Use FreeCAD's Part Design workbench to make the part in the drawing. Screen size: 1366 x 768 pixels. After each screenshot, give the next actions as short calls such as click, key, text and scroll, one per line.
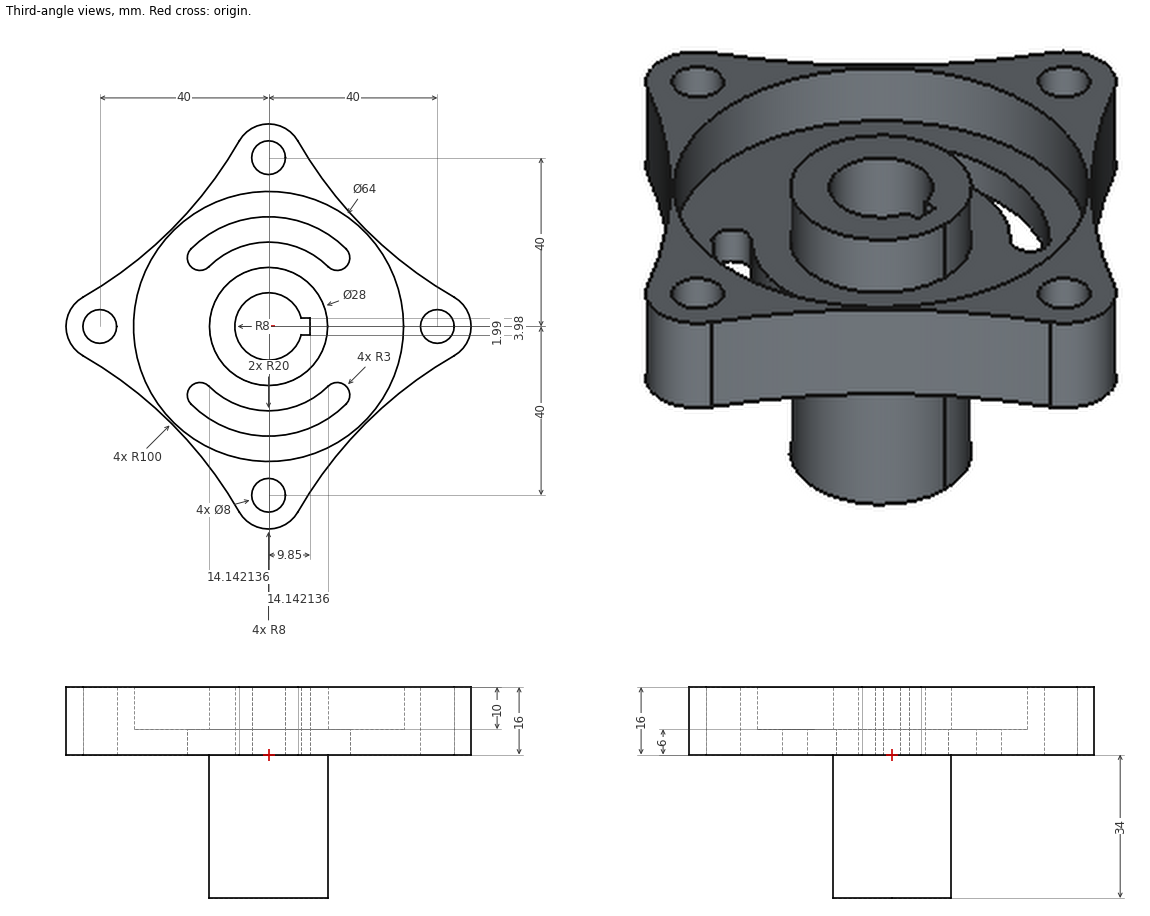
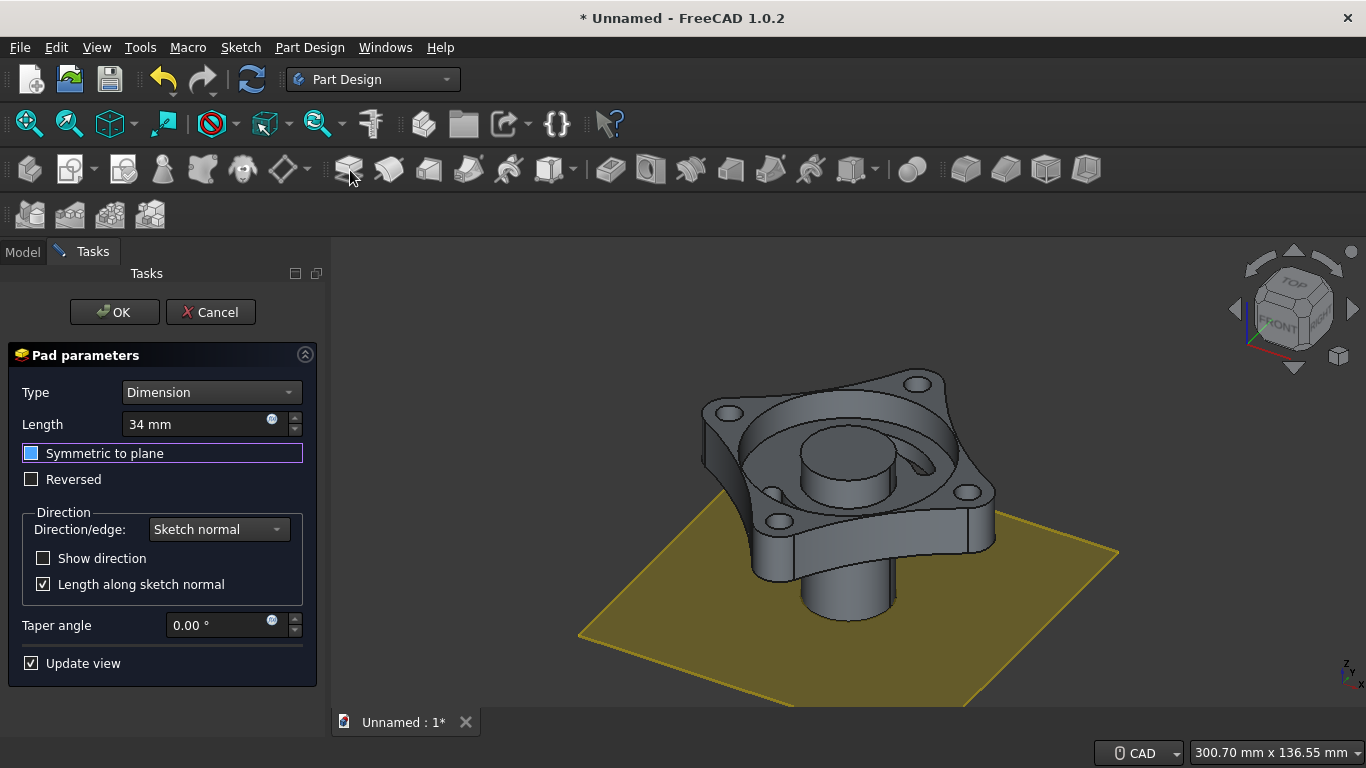
click(115, 312)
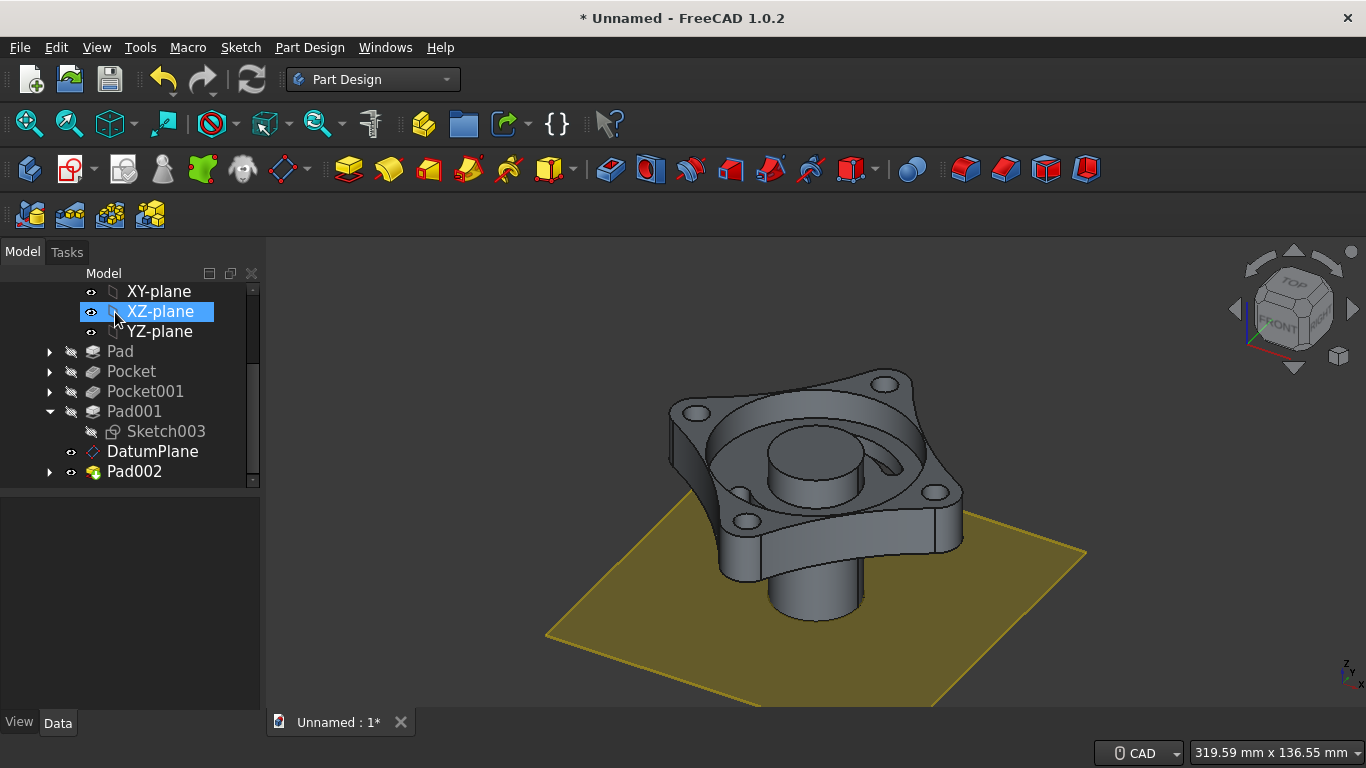
click(116, 452)
key(space)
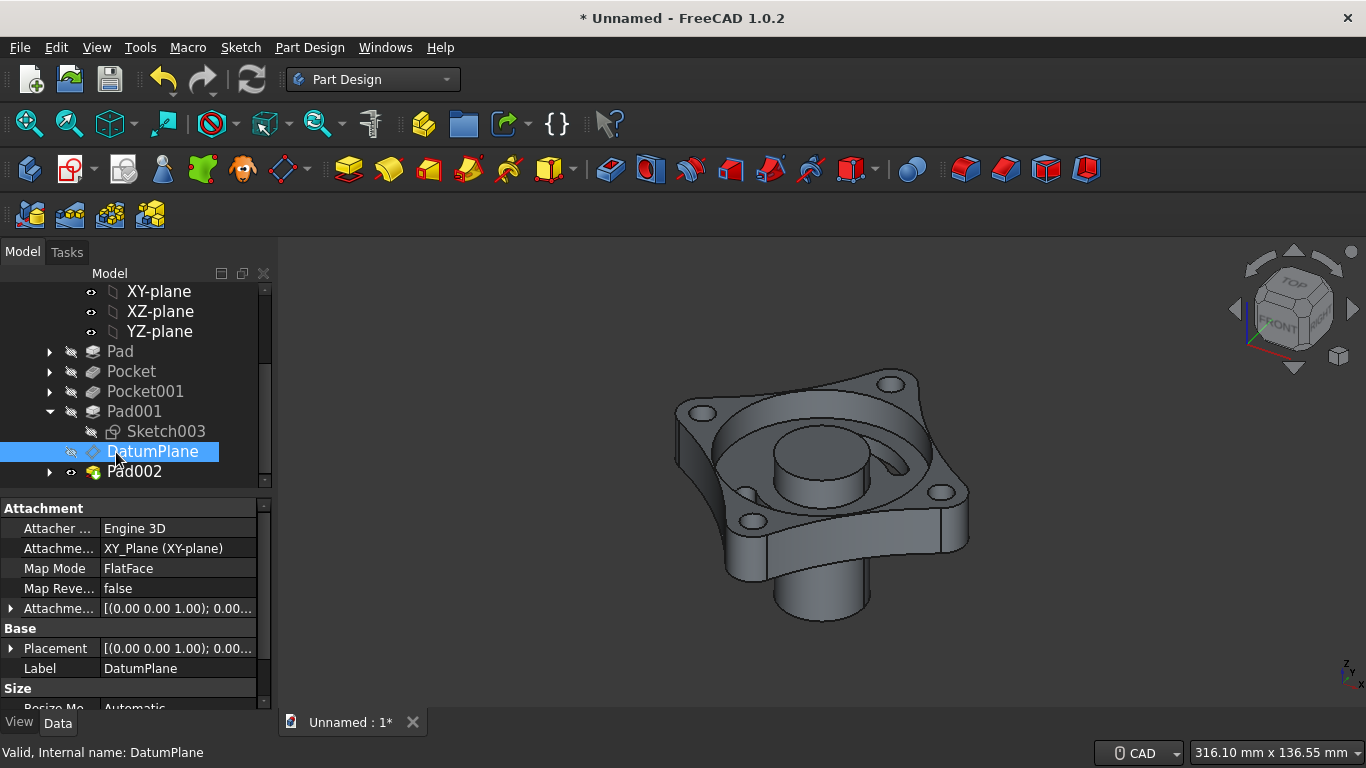
click(30, 124)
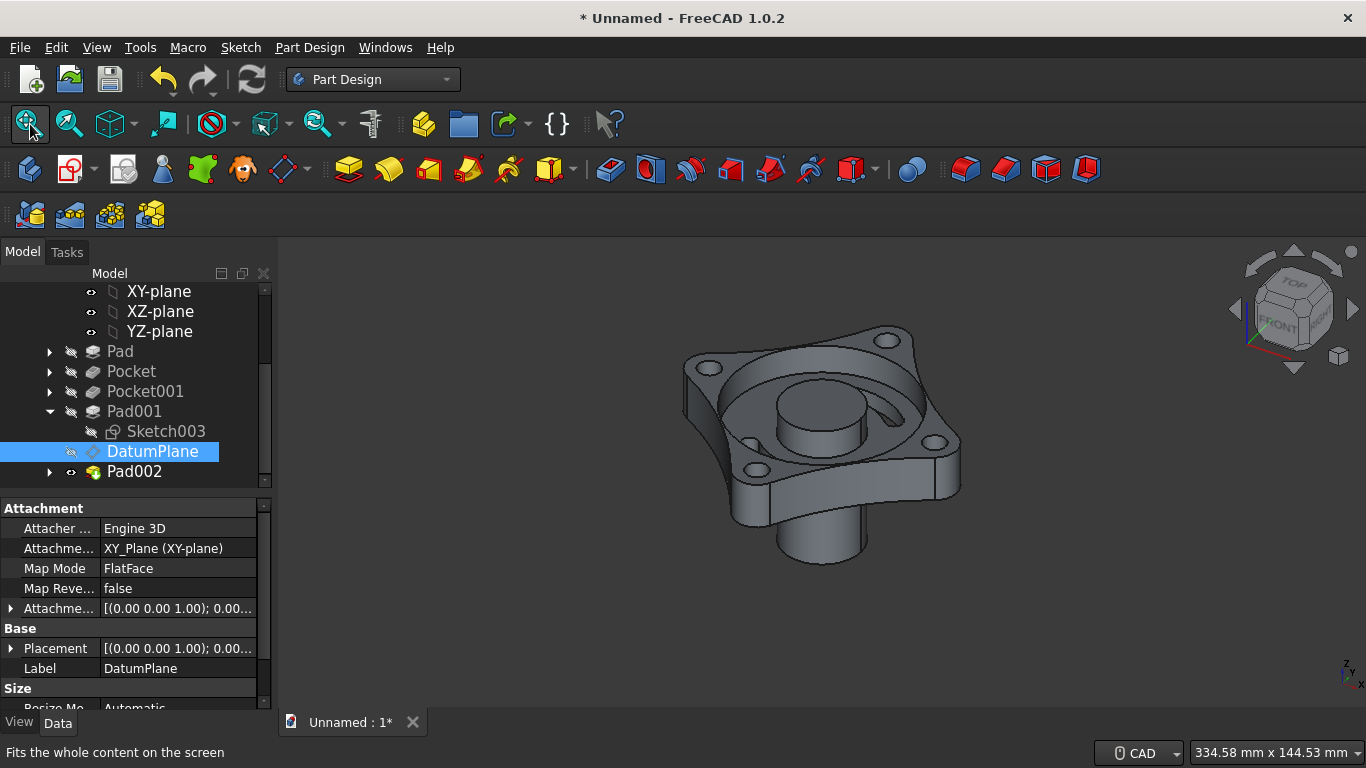
key(0)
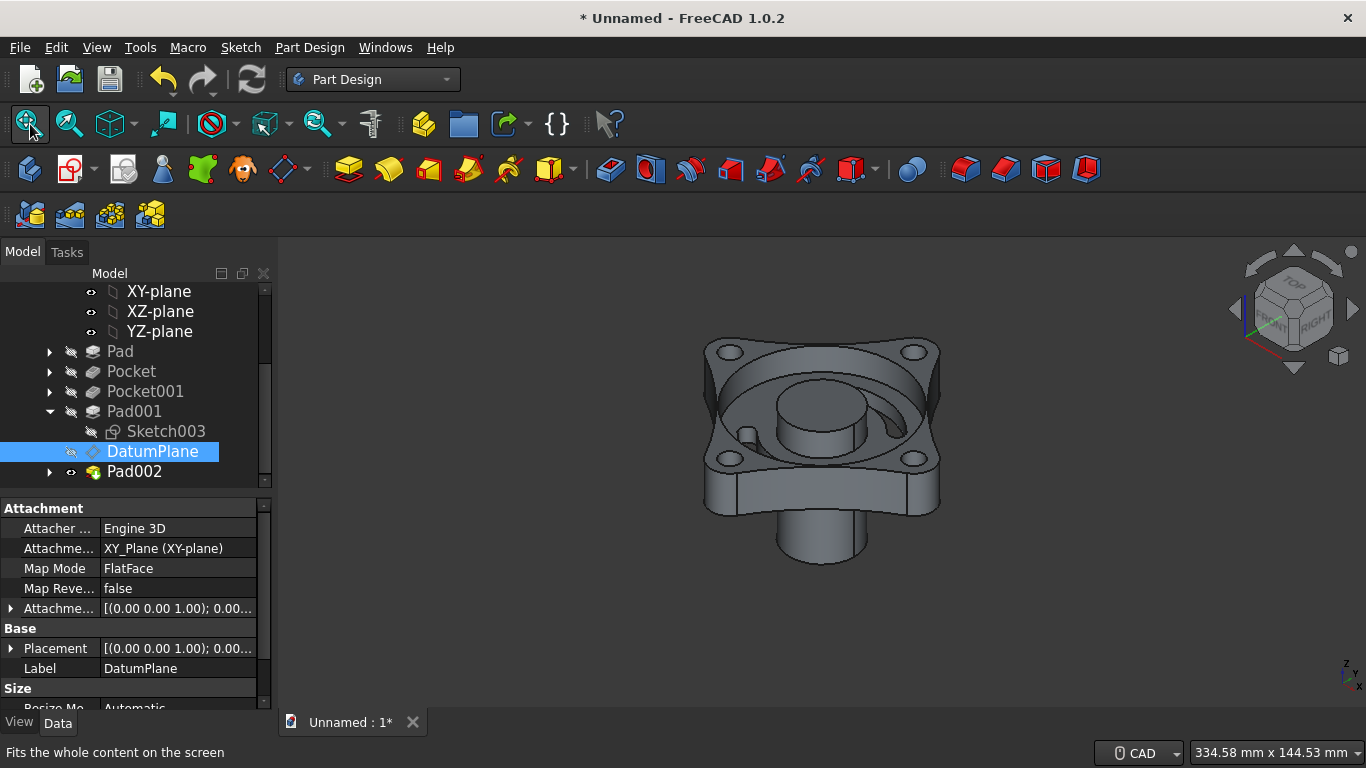
key(2)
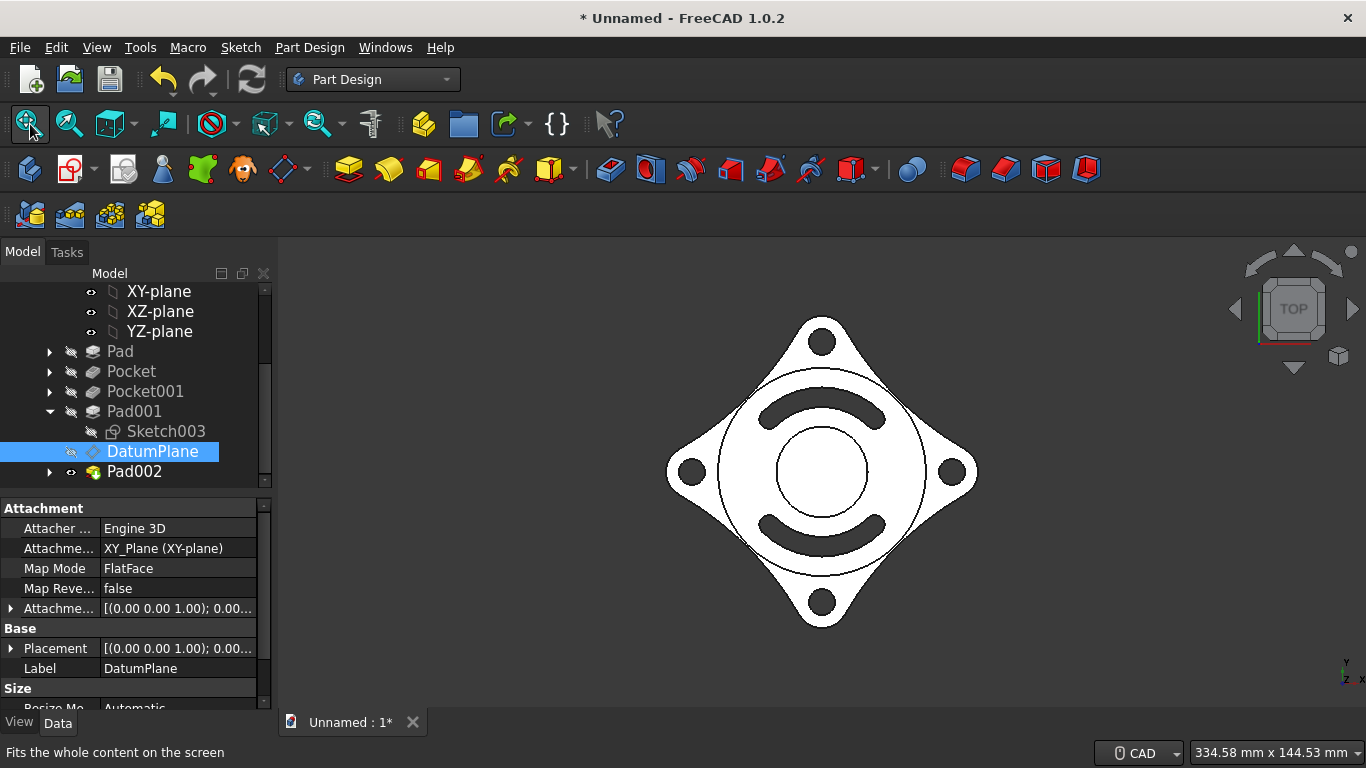
click(940, 450)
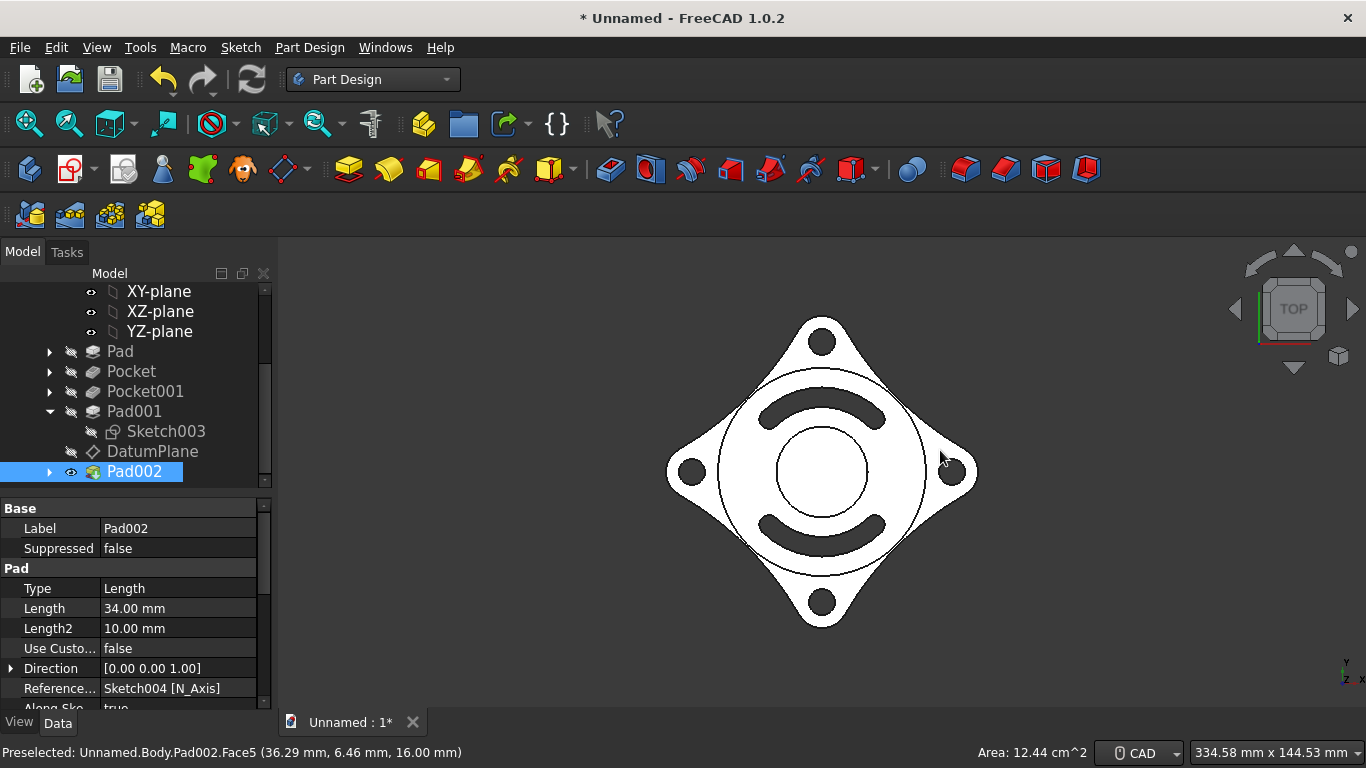
click(70, 170)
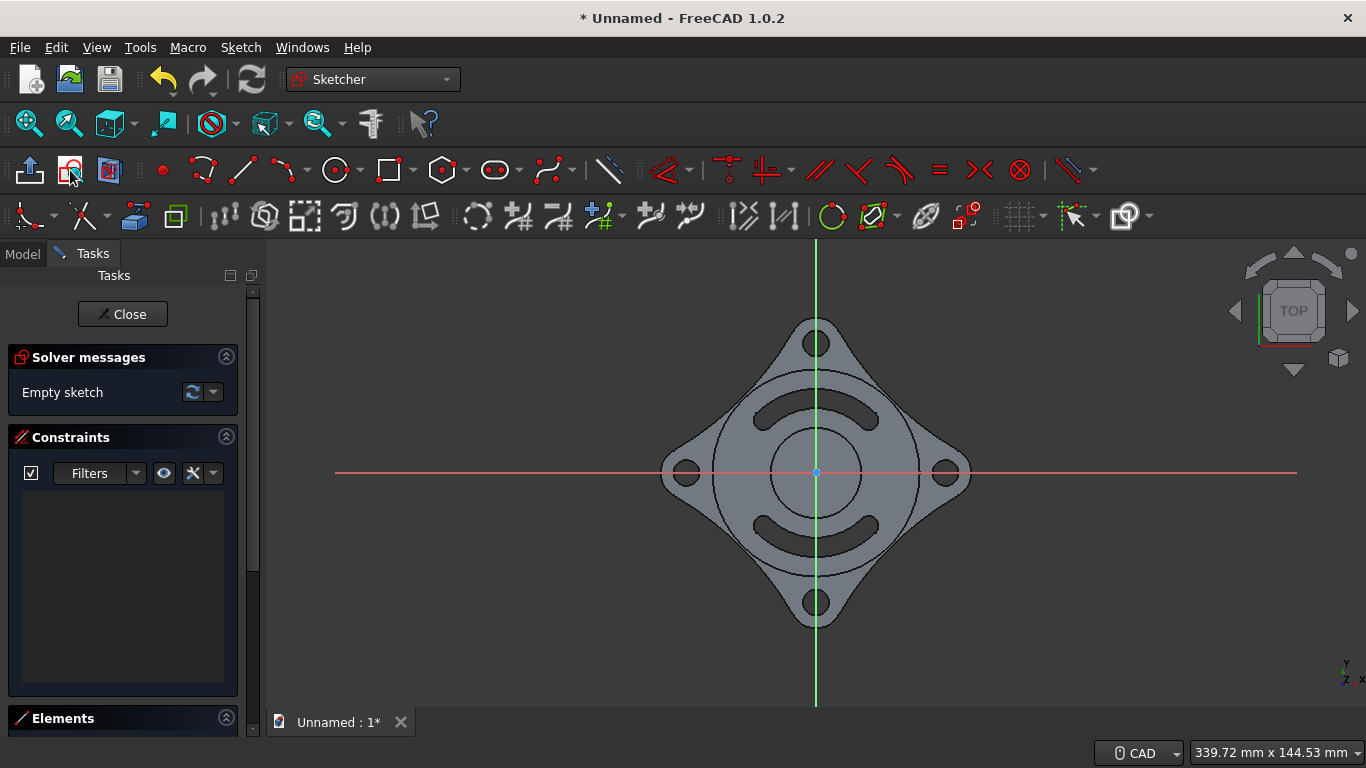
scroll(826, 473, up, 12)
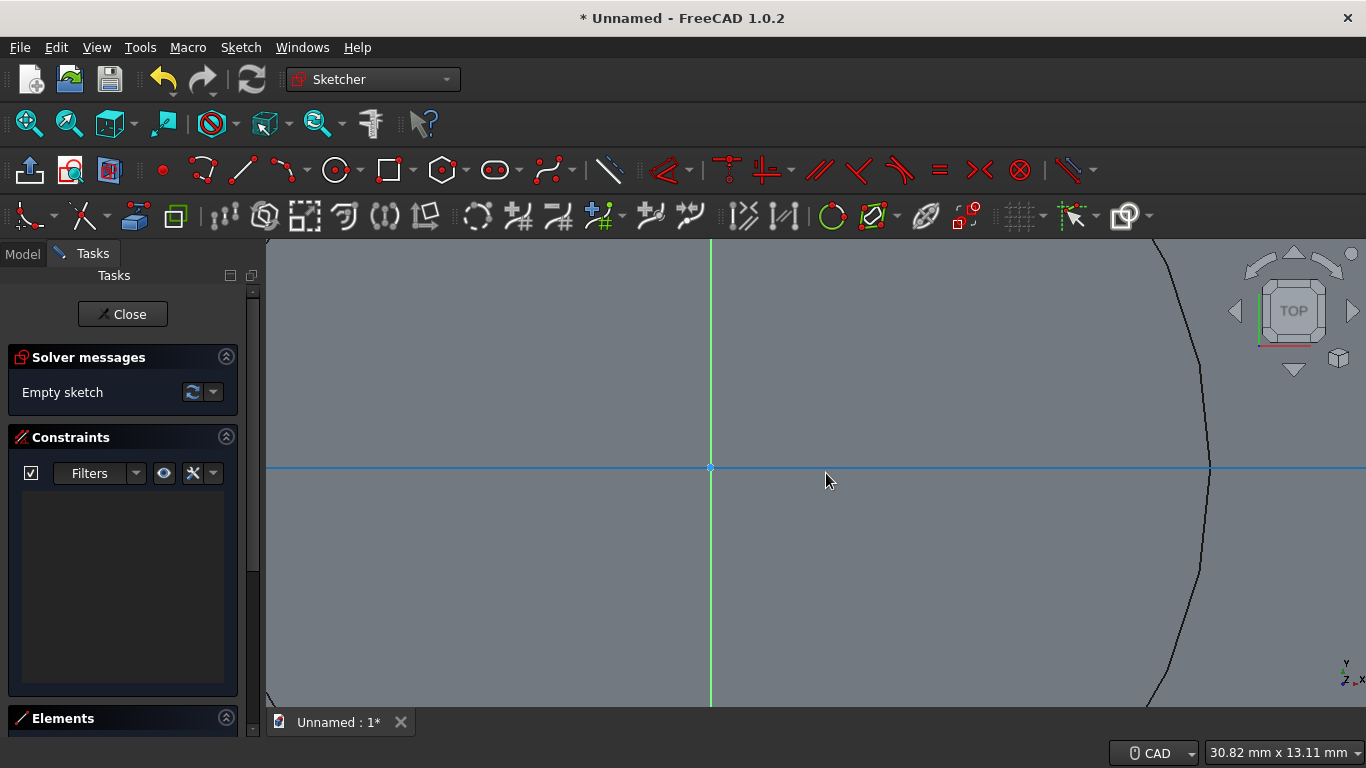
key(g)
key(m)